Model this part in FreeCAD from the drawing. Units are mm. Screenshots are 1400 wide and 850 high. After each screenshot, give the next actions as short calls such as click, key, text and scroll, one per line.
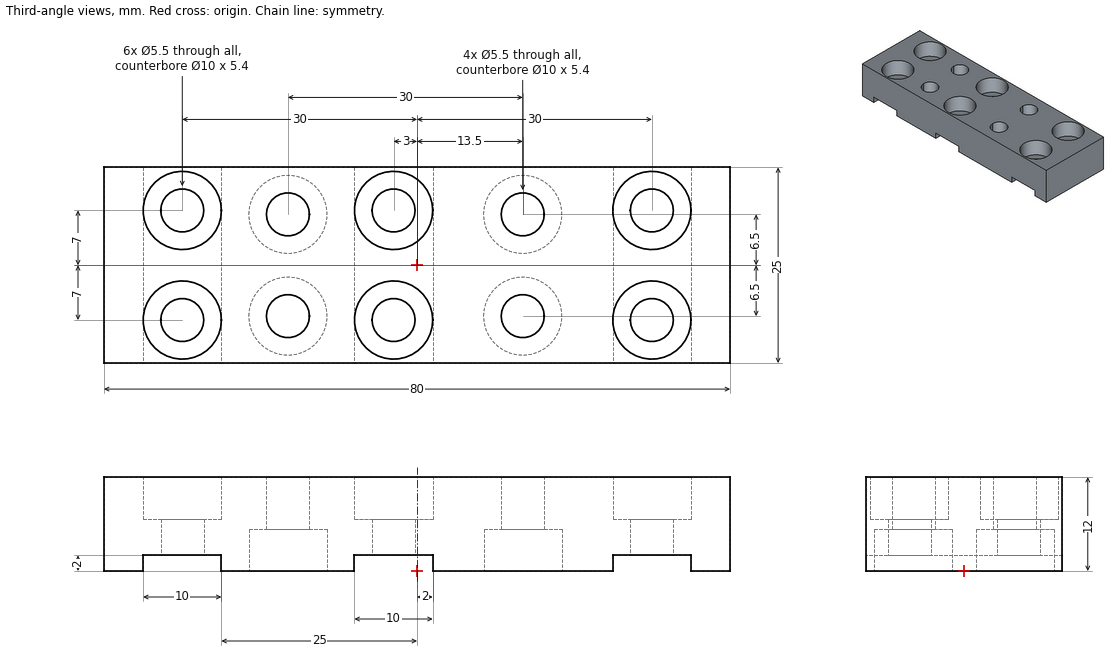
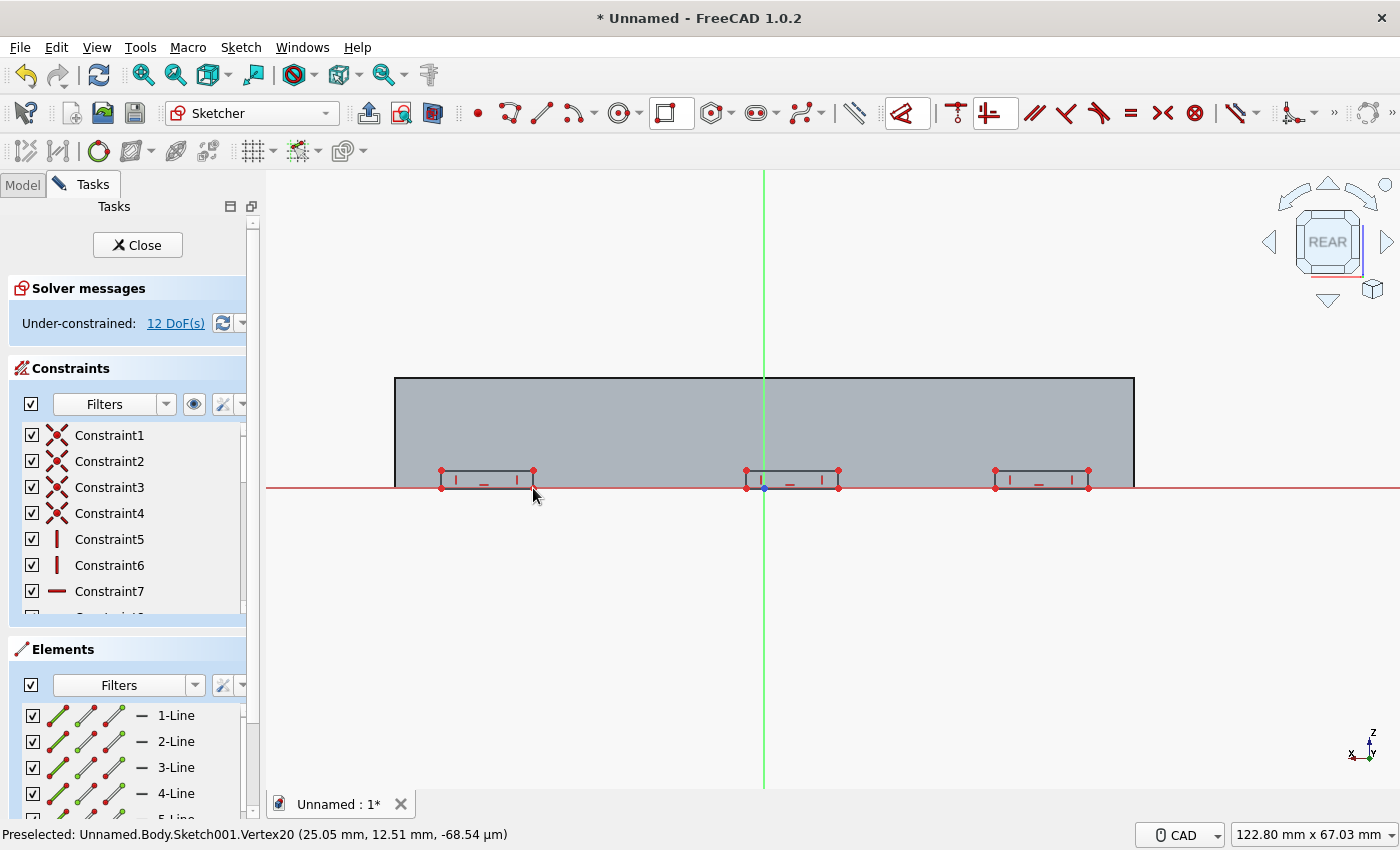
click(1088, 471)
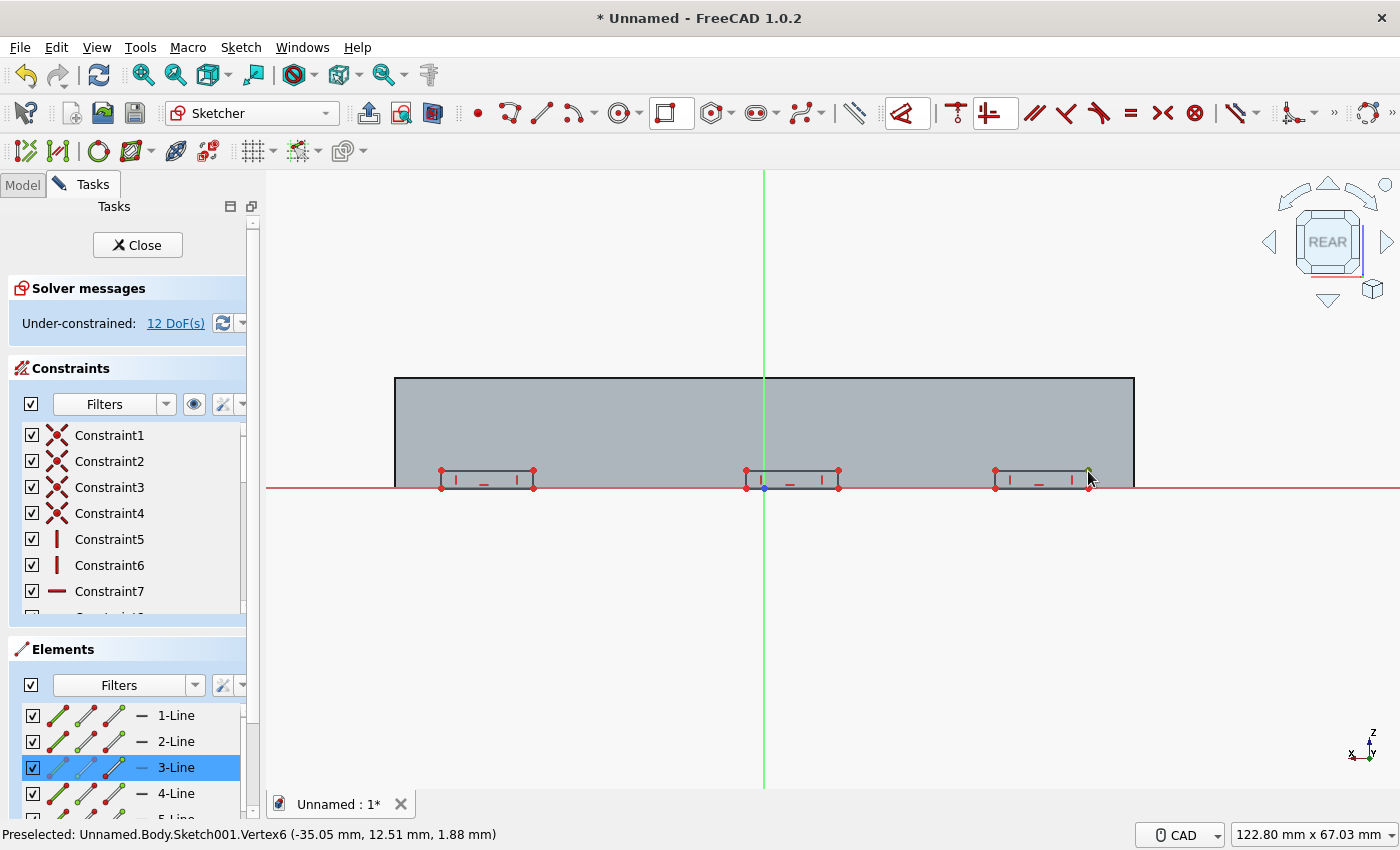
click(441, 471)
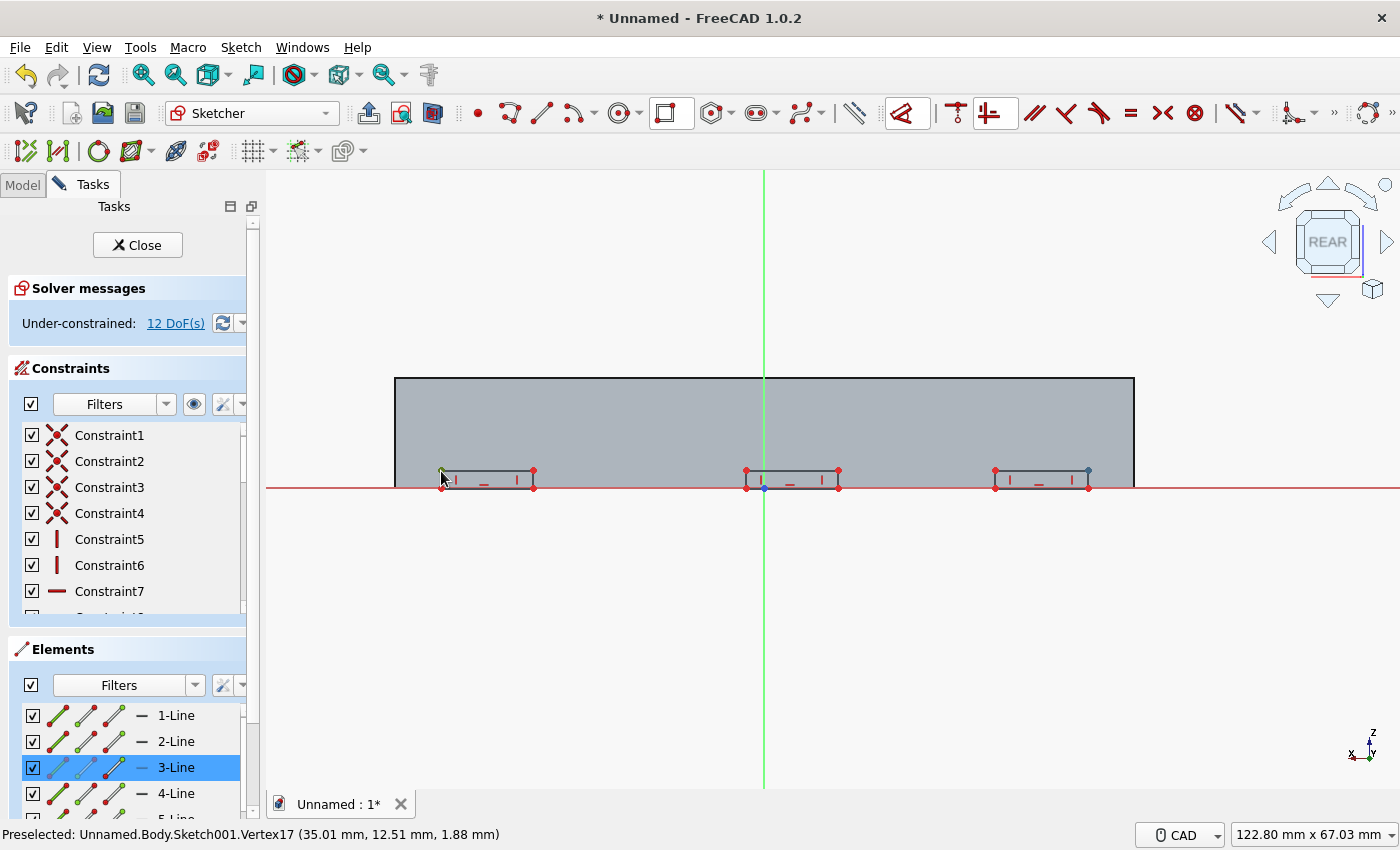
click(764, 721)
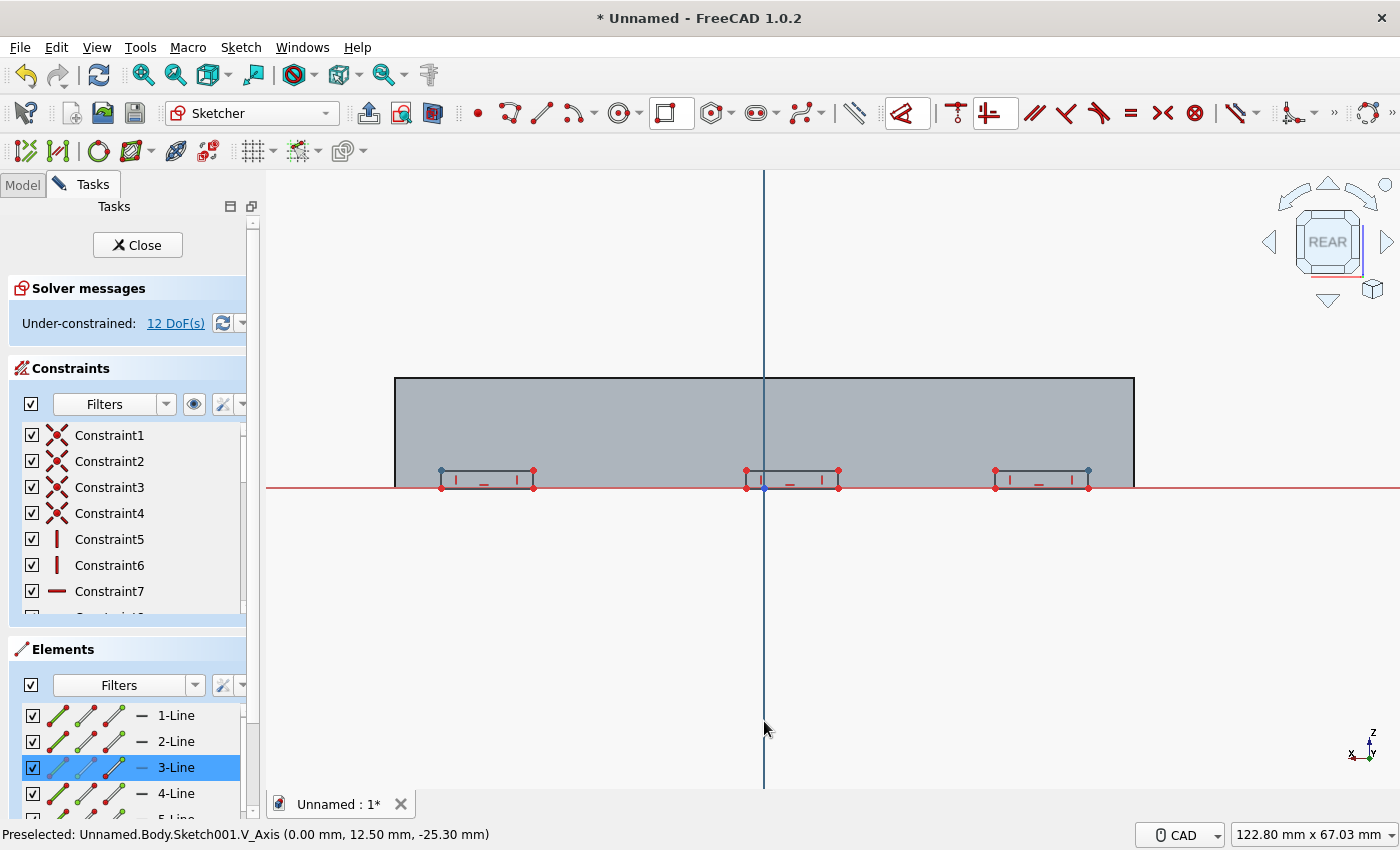
click(1164, 114)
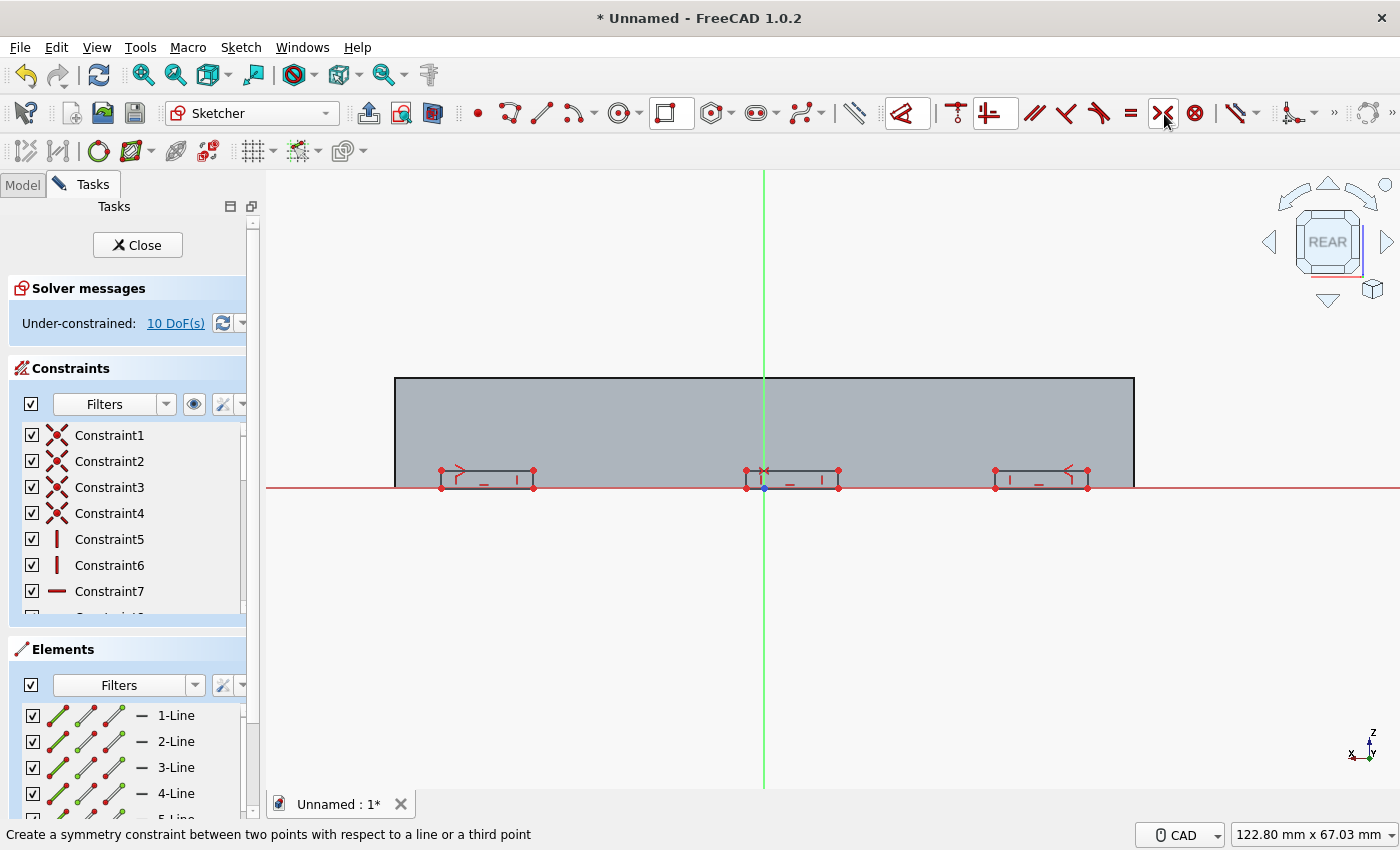
click(995, 489)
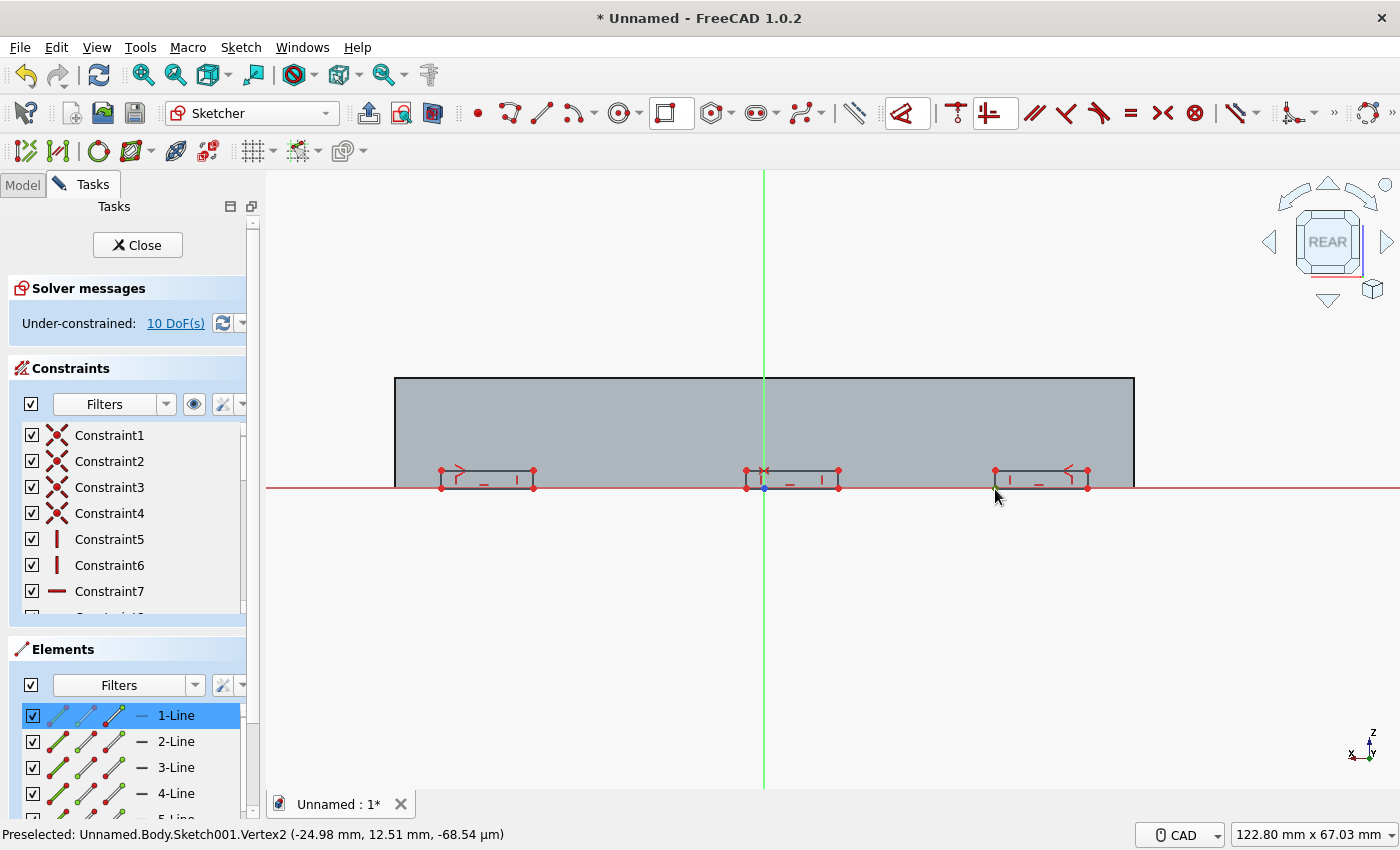
click(533, 489)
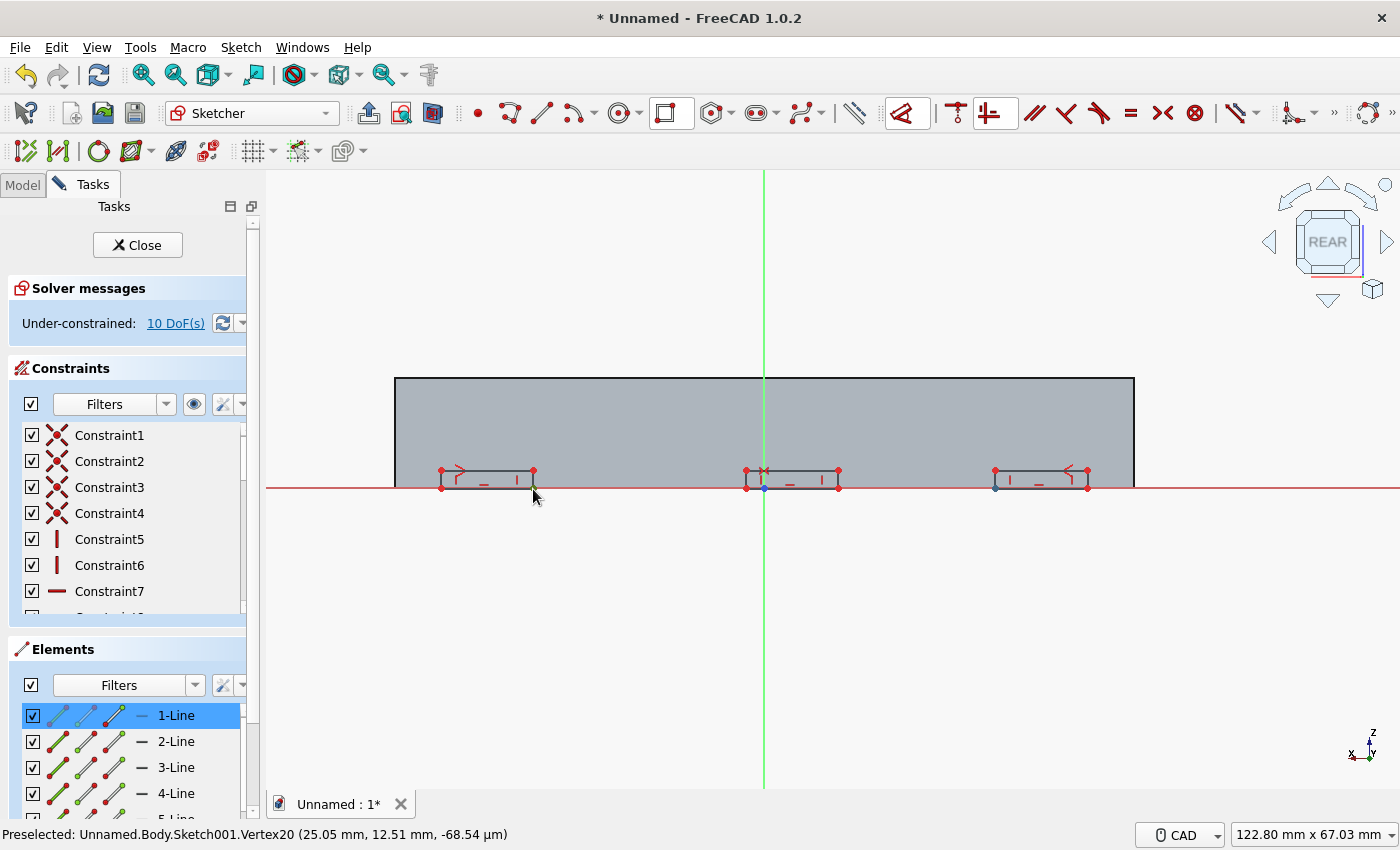
click(764, 721)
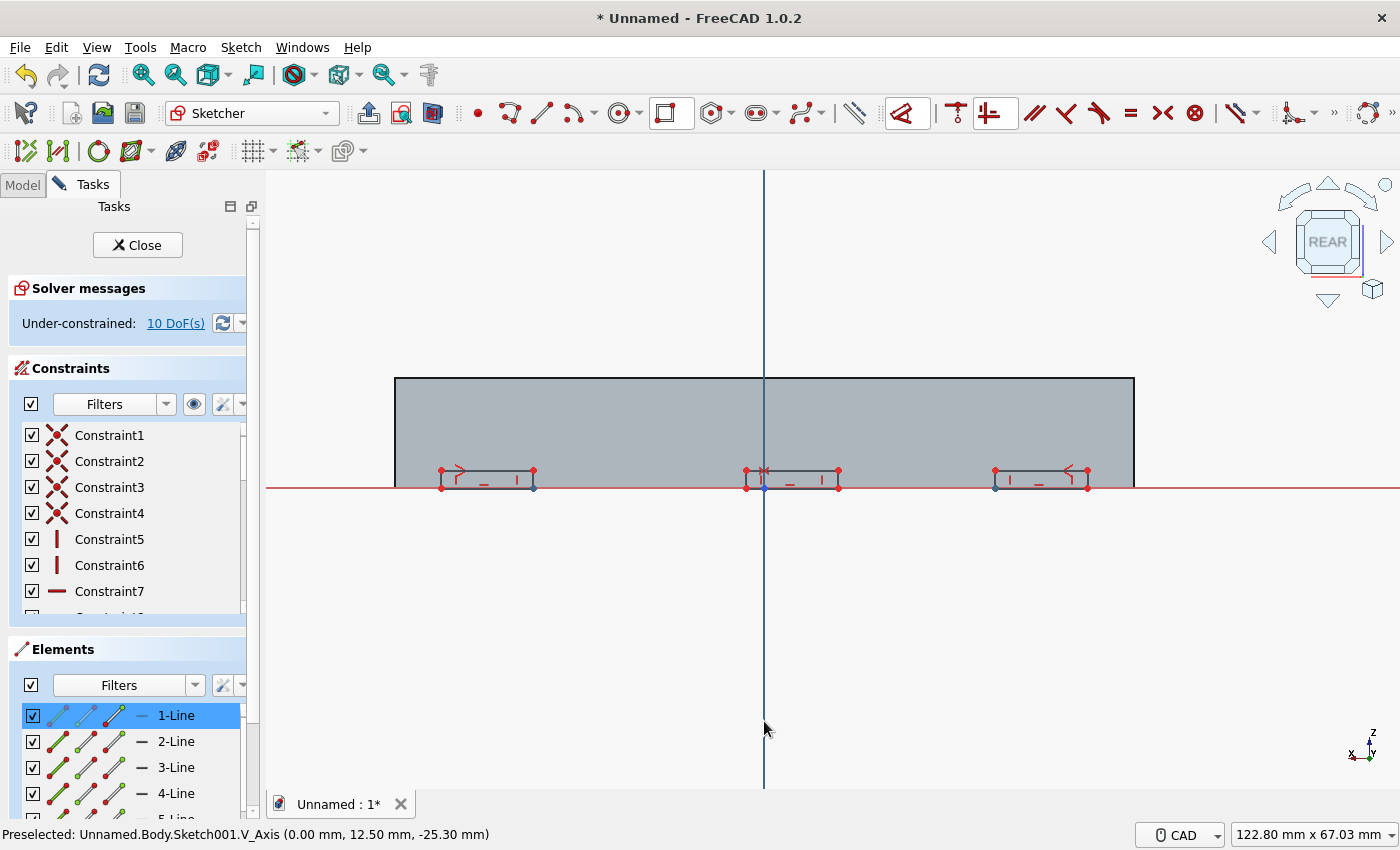
click(1164, 114)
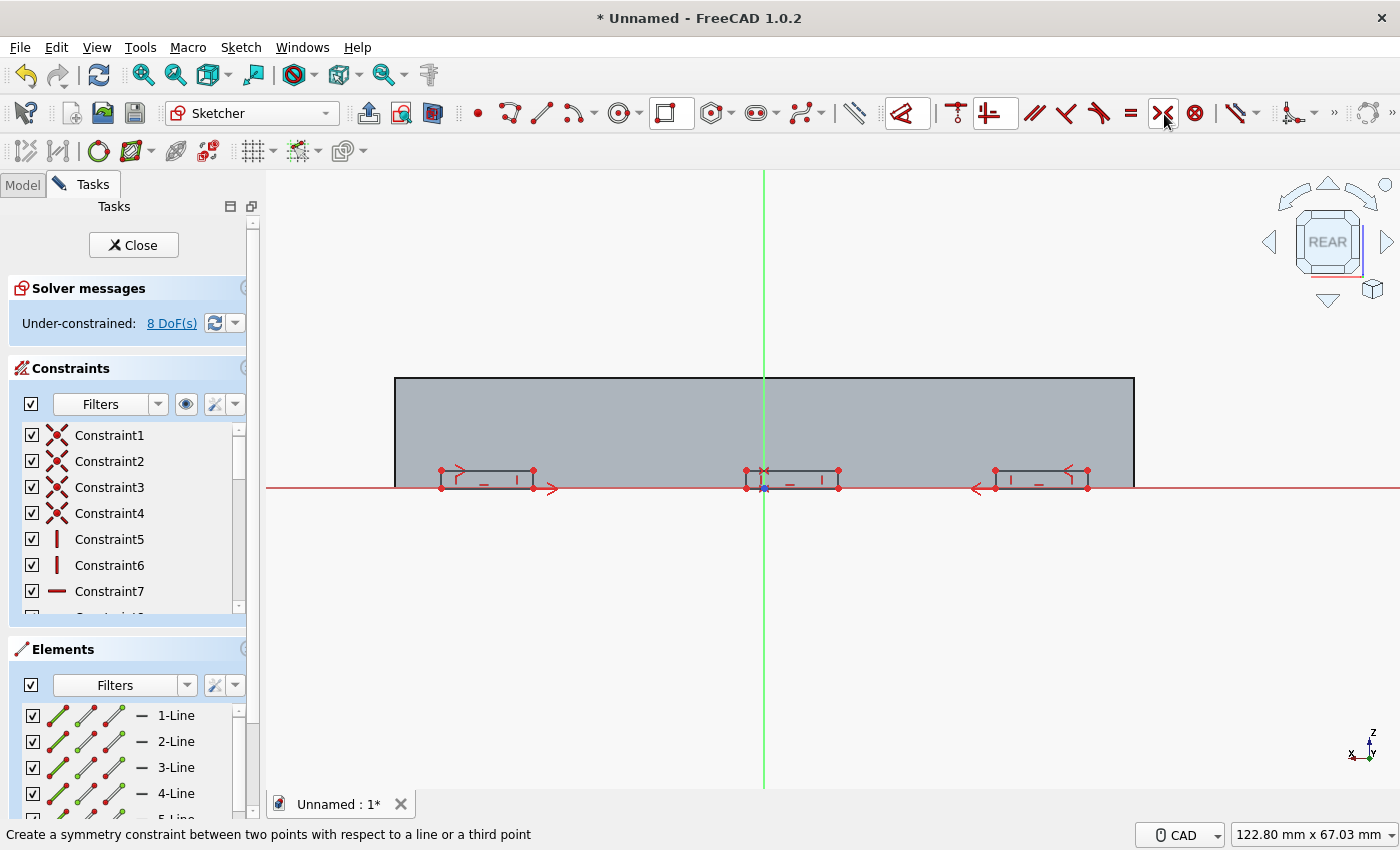
click(996, 489)